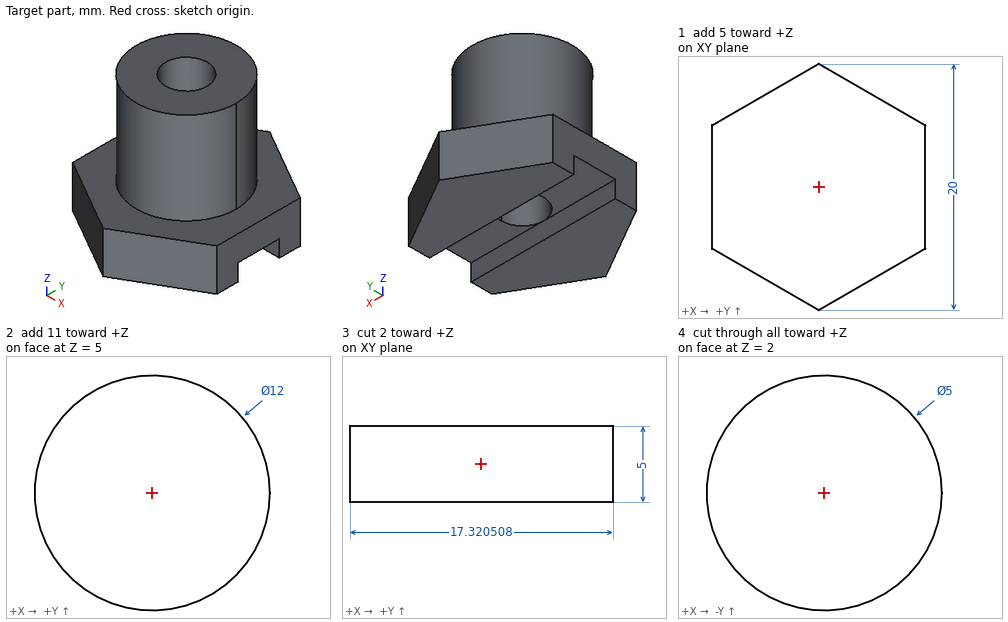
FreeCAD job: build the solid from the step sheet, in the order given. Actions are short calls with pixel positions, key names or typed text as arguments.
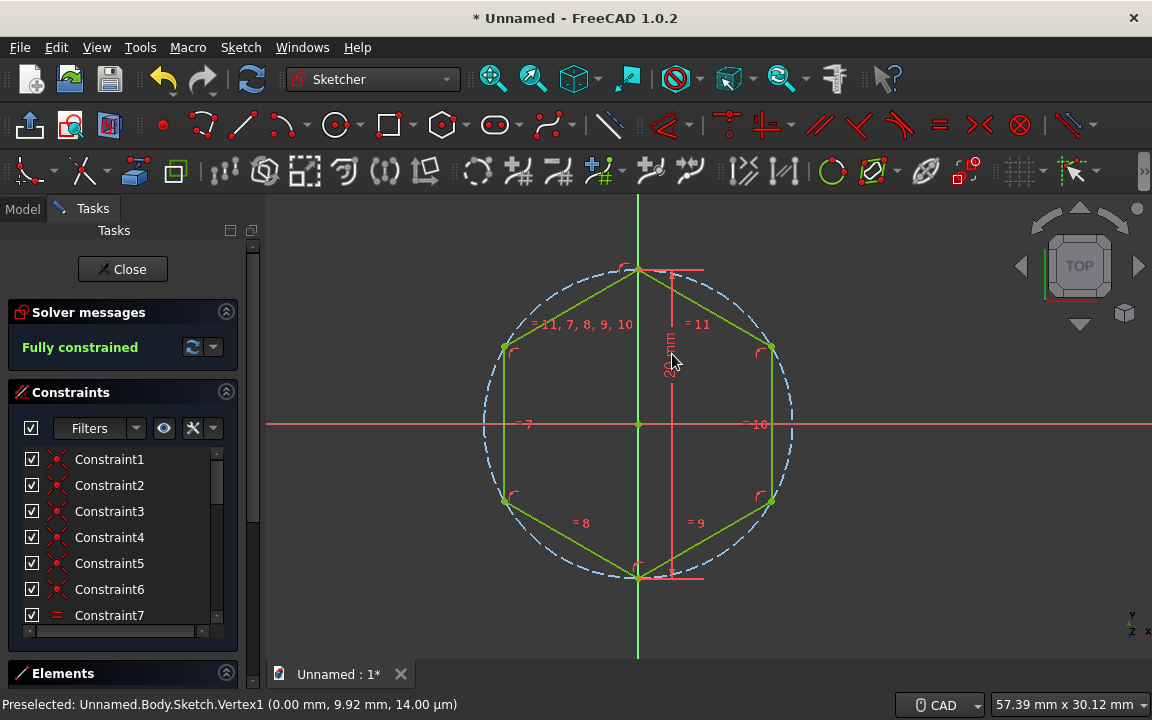
click(123, 269)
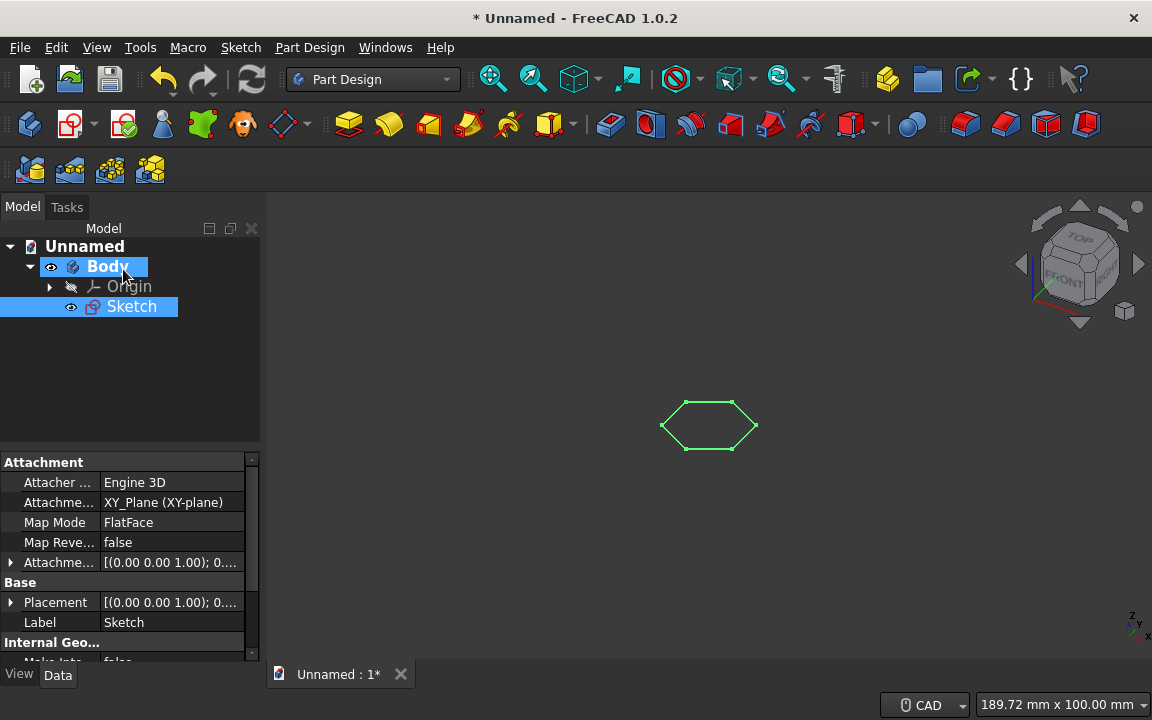
click(350, 124)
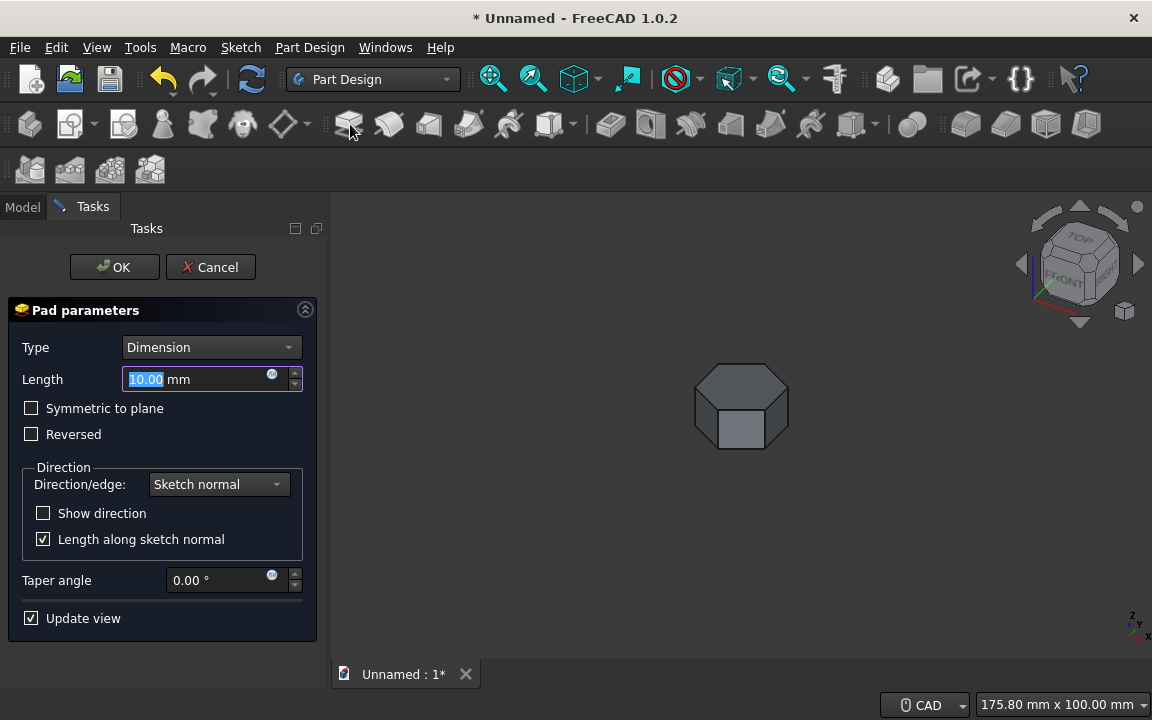
text(5)
key(Tab)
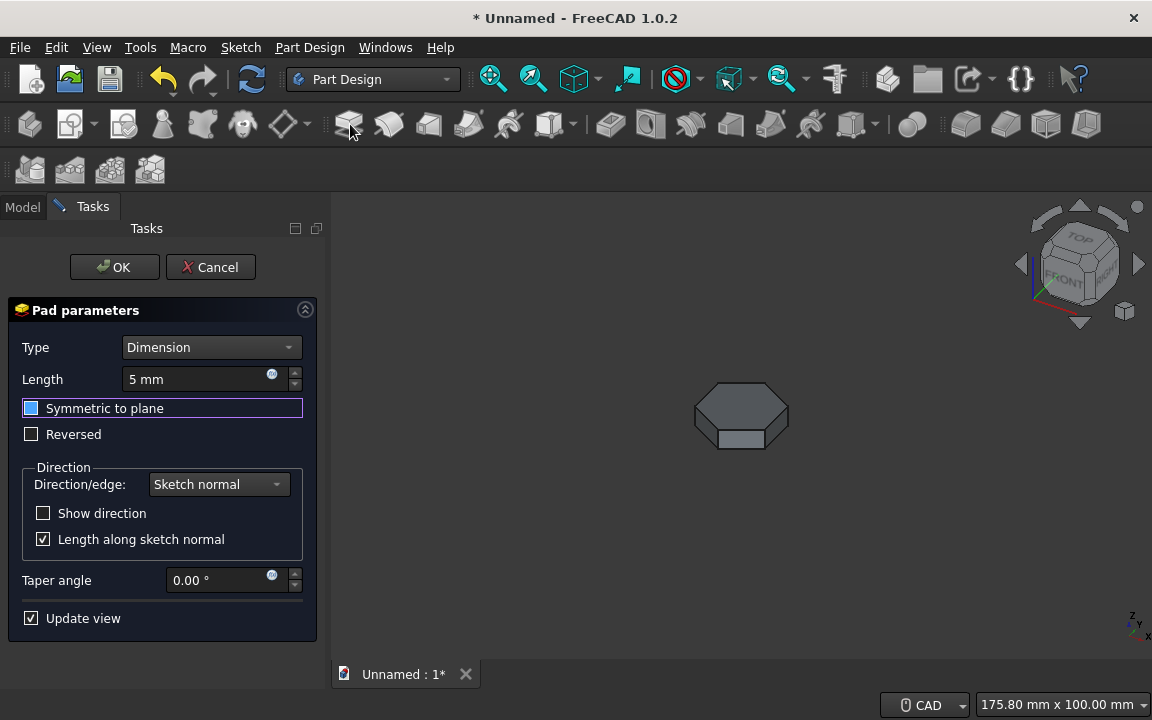
click(115, 267)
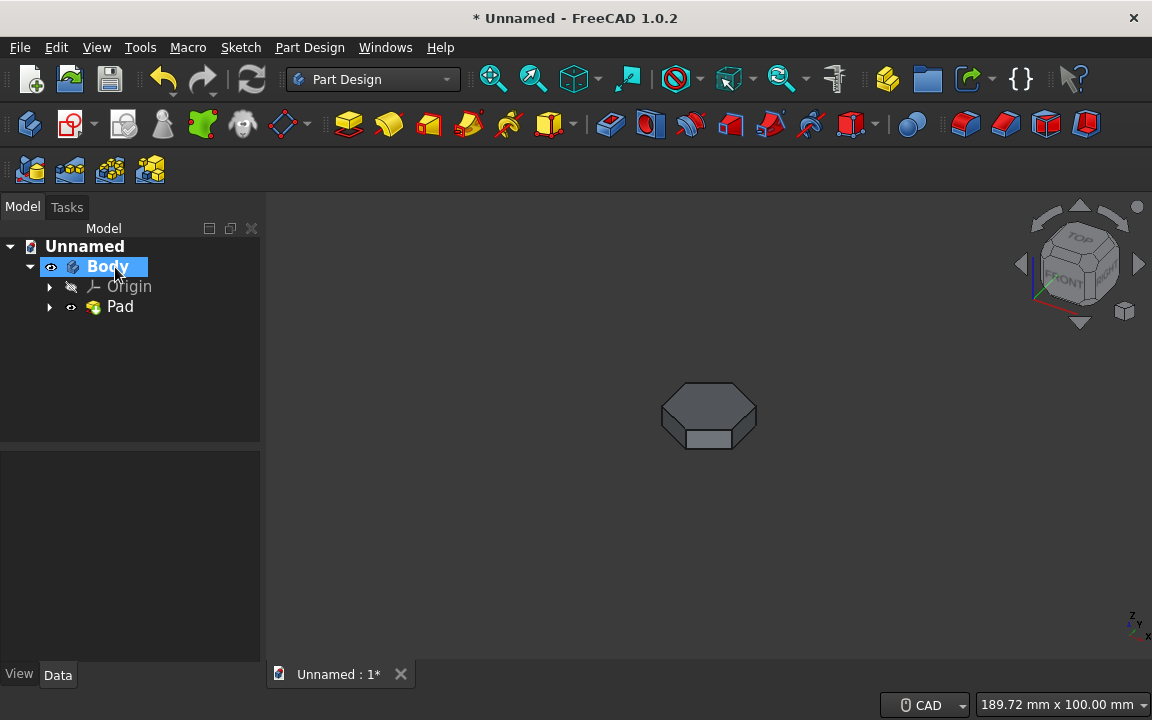
key(v)
key(f)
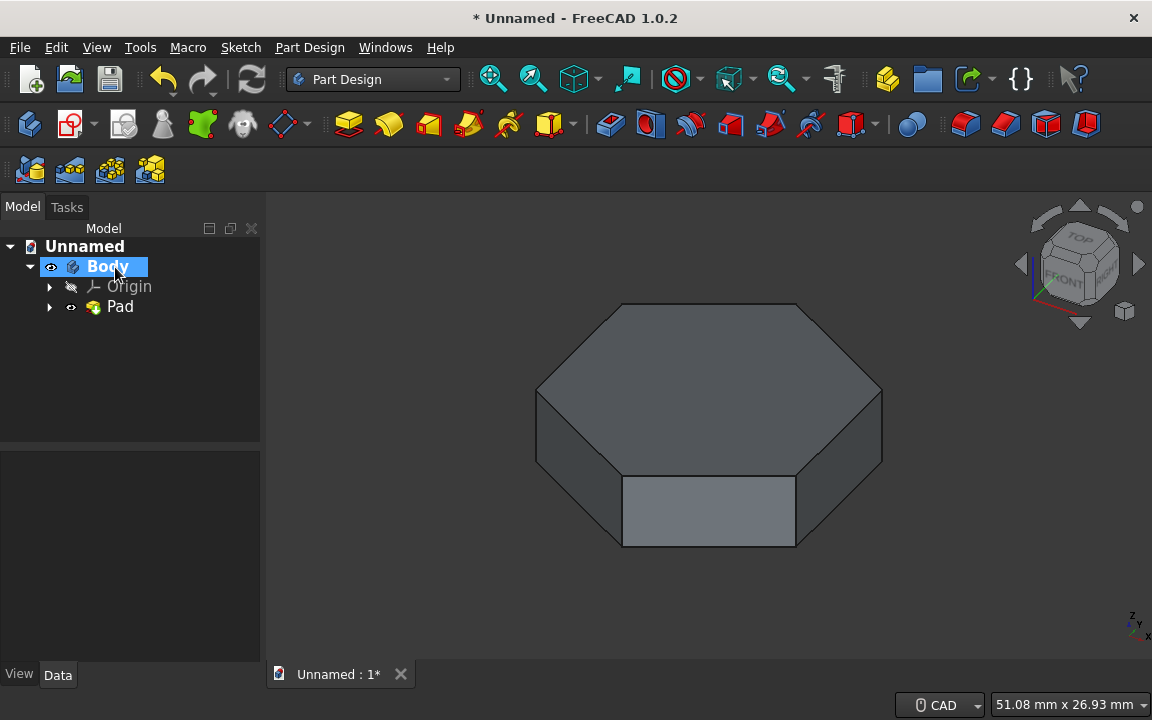
click(709, 389)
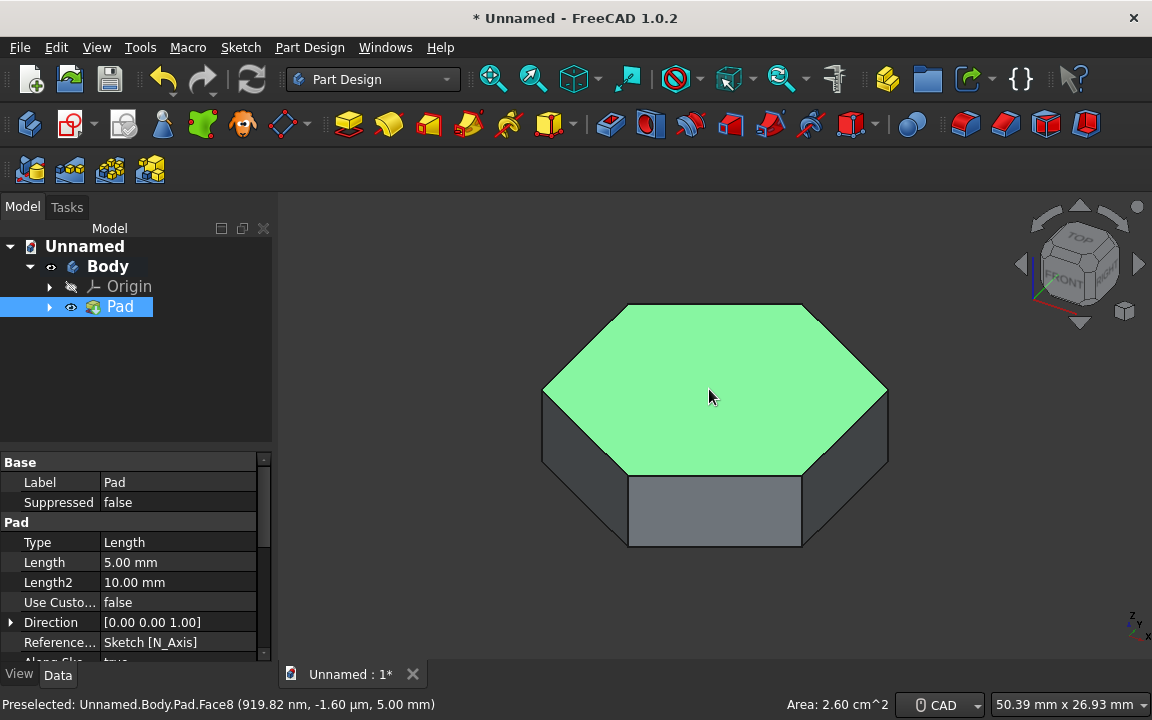
click(70, 124)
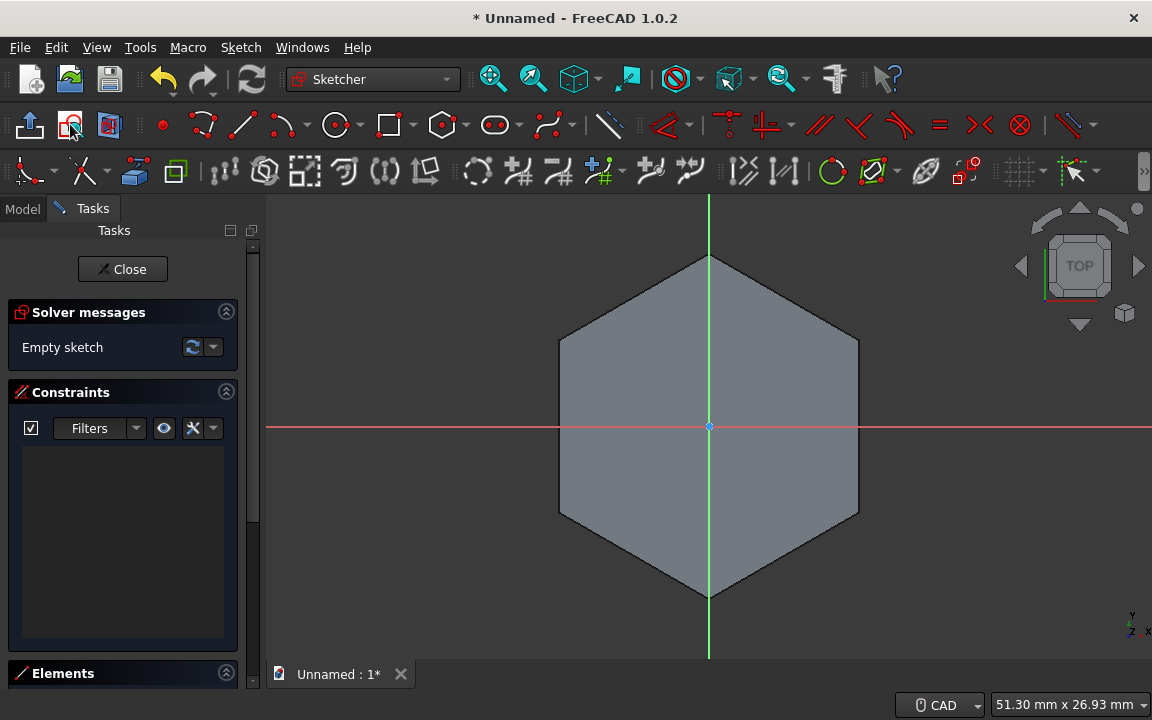
scroll(848, 426, up, 2)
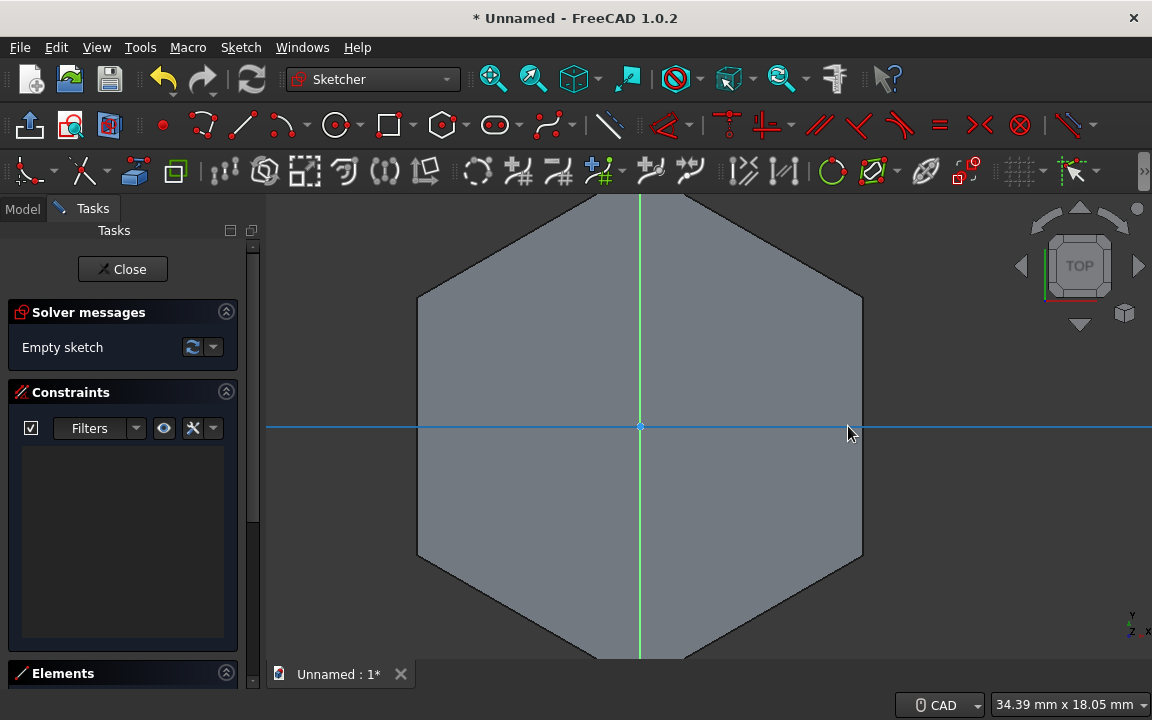
key(g)
key(c)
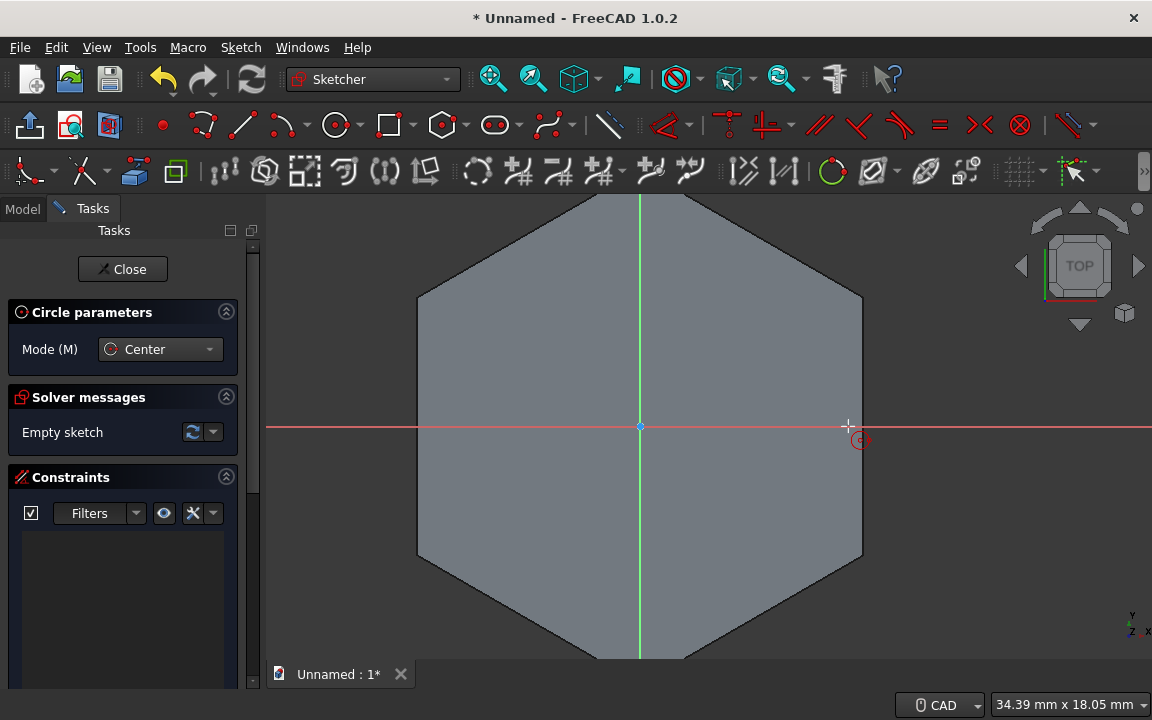
click(640, 426)
click(750, 317)
key(Escape)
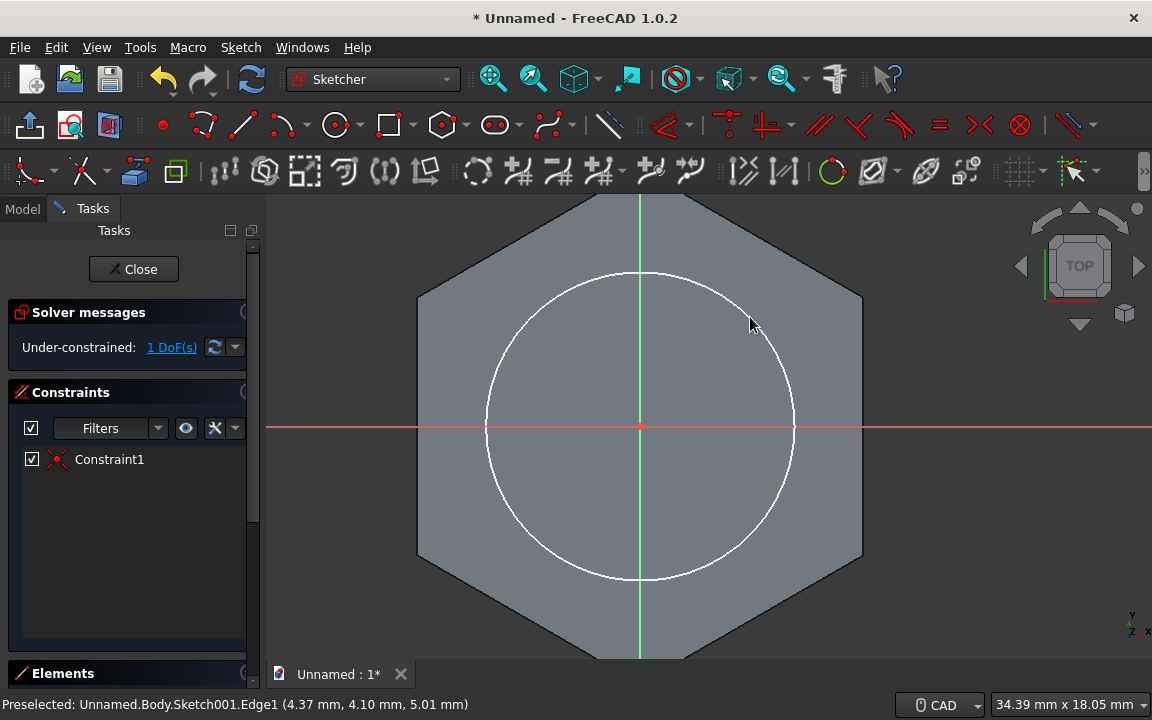
key(d)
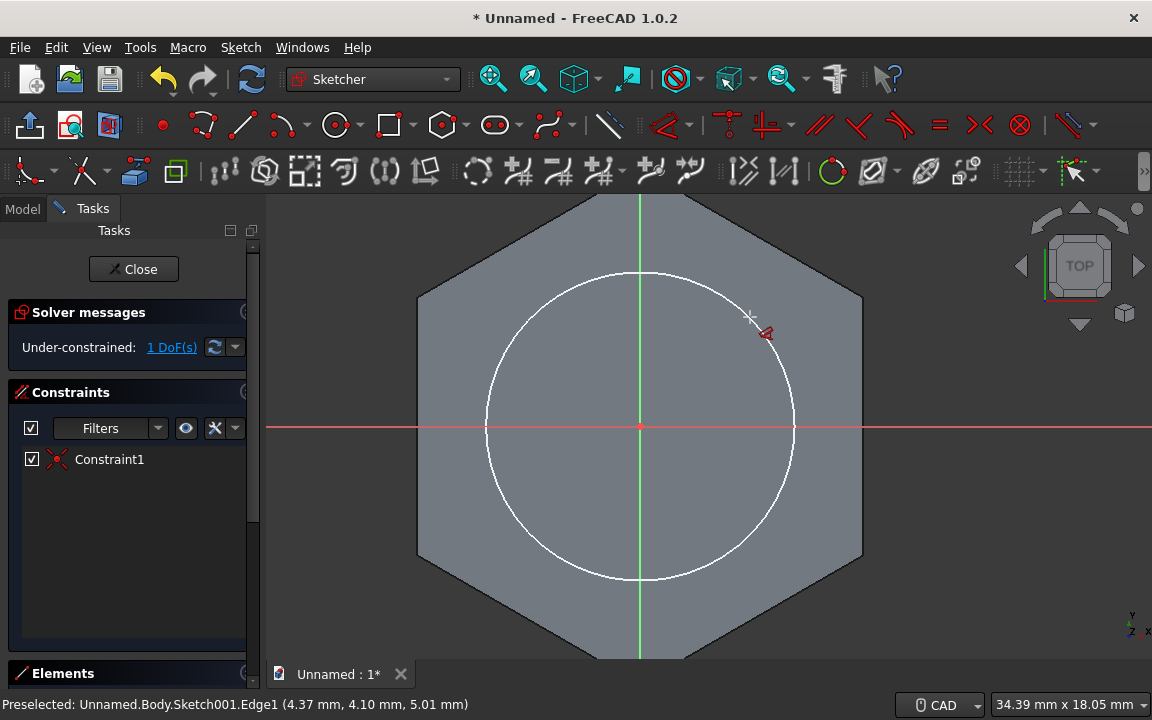
click(749, 317)
click(772, 294)